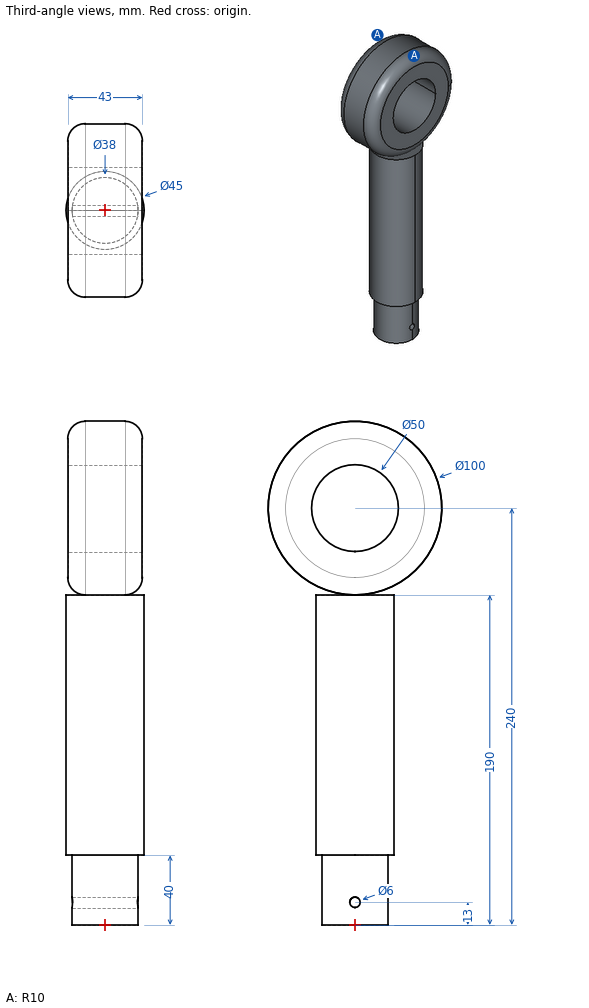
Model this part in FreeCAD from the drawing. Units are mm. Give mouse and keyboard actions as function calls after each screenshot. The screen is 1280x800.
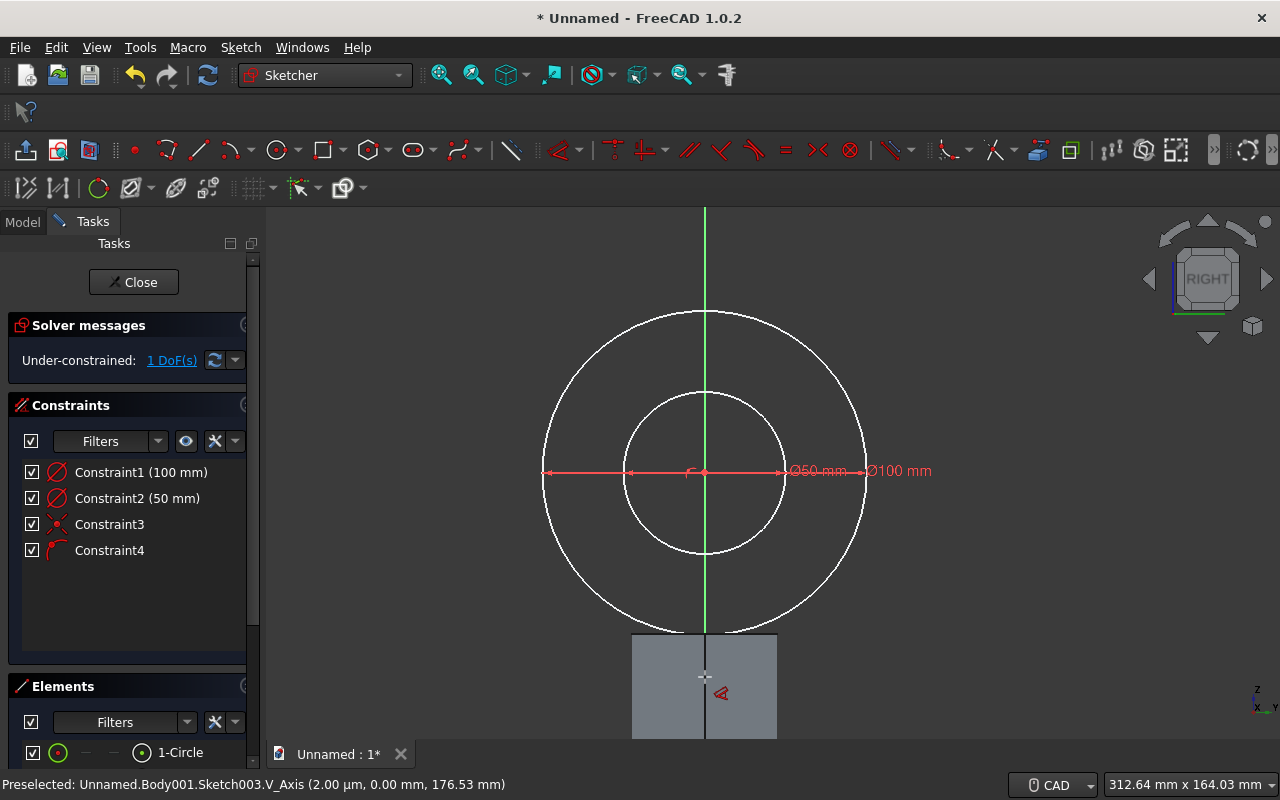
click(705, 473)
click(739, 592)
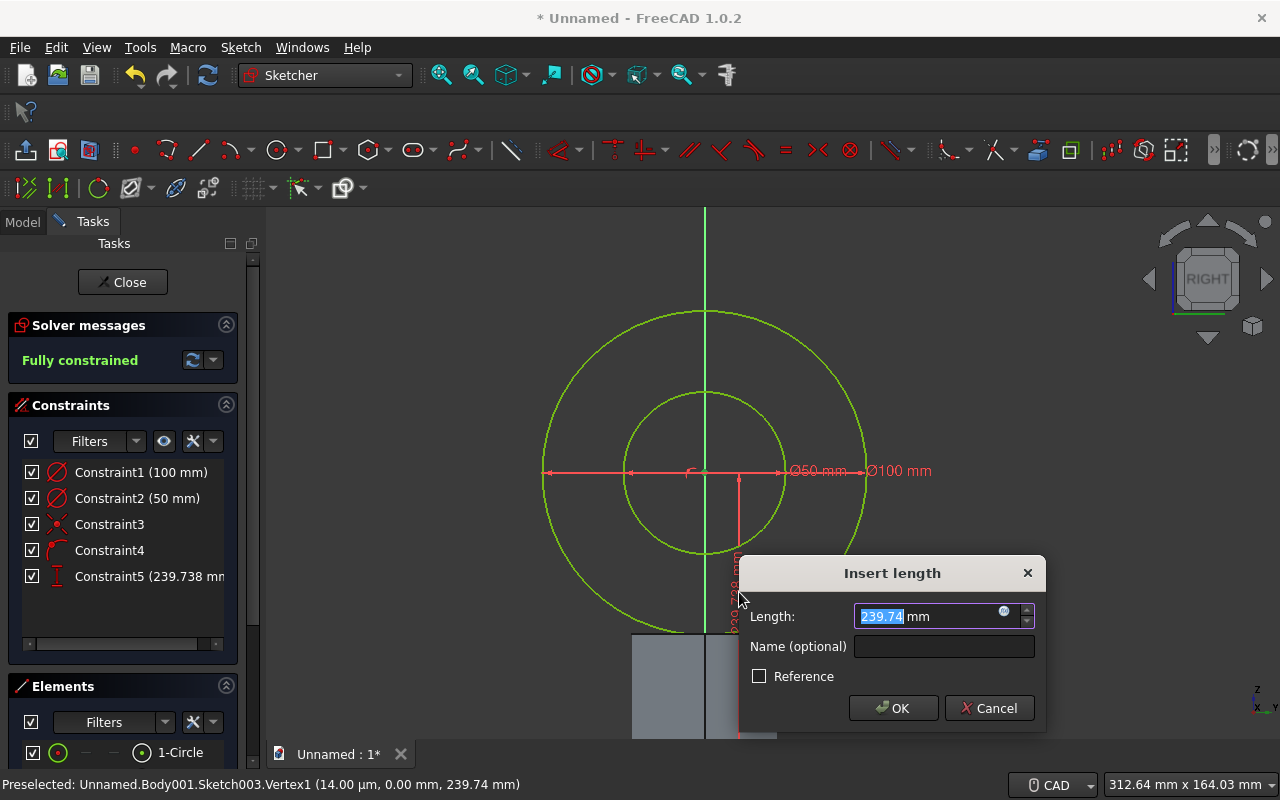
text(240)
key(Return)
key(Escape)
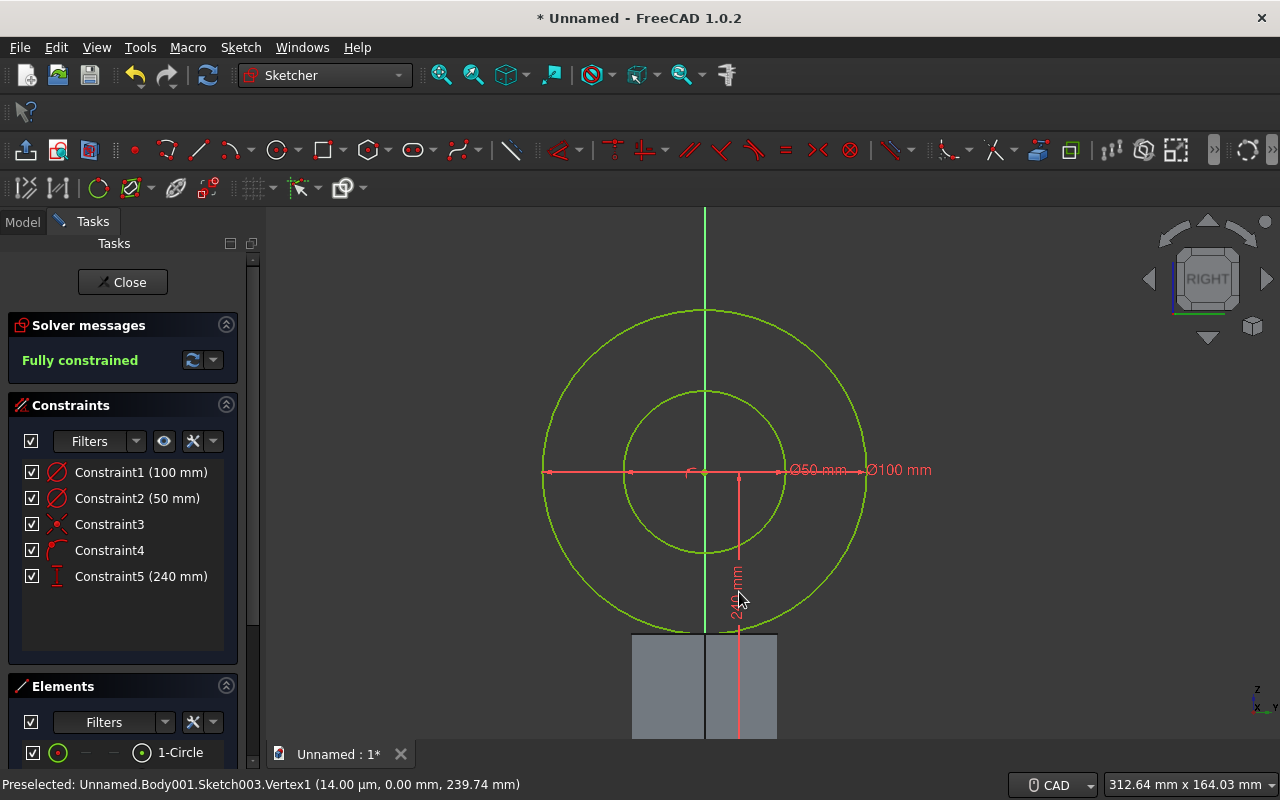
click(123, 282)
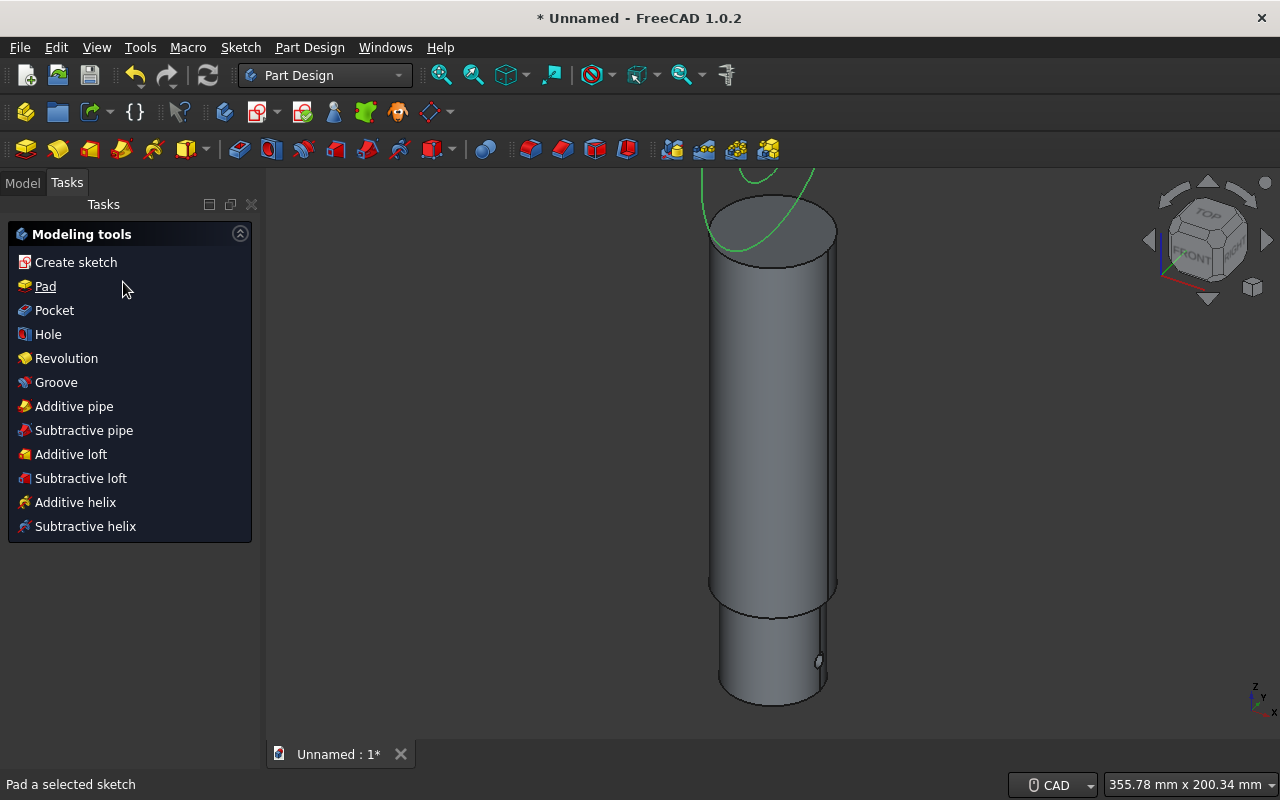
click(26, 150)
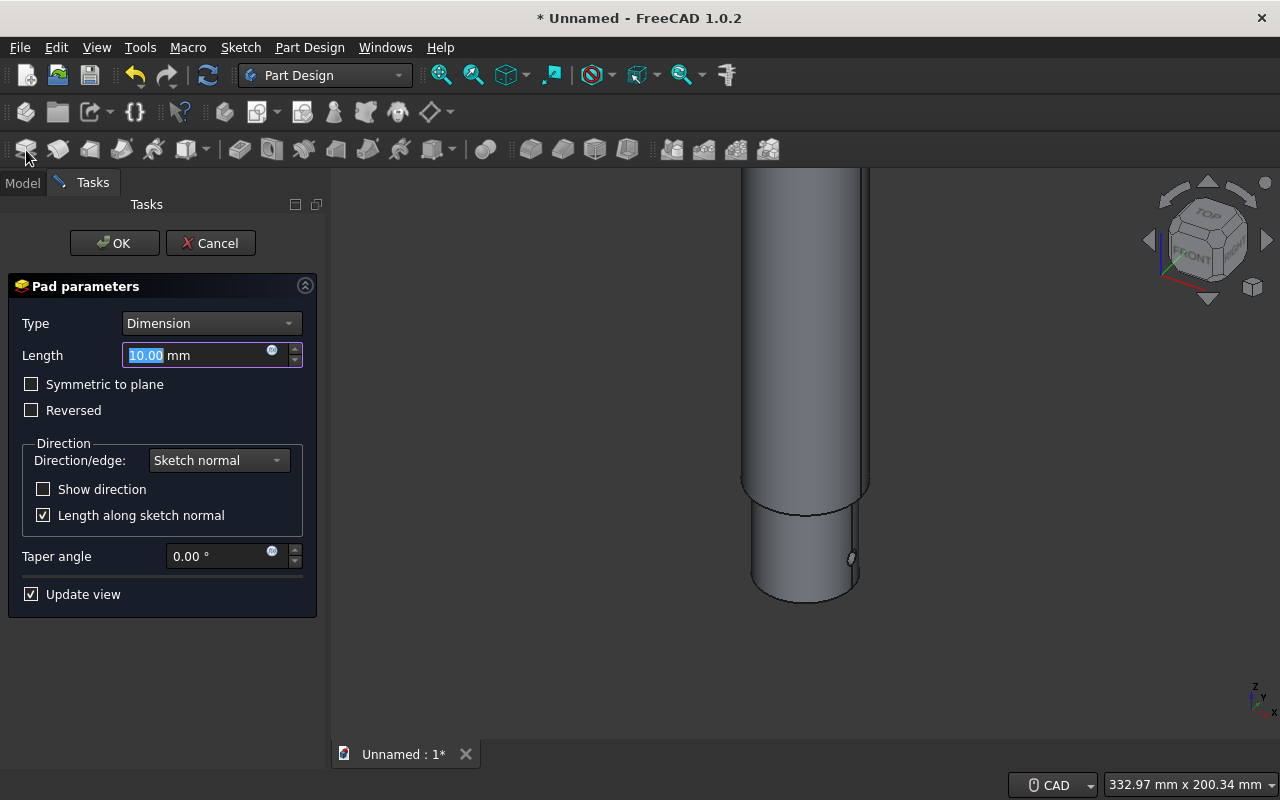
text(43)
key(Tab)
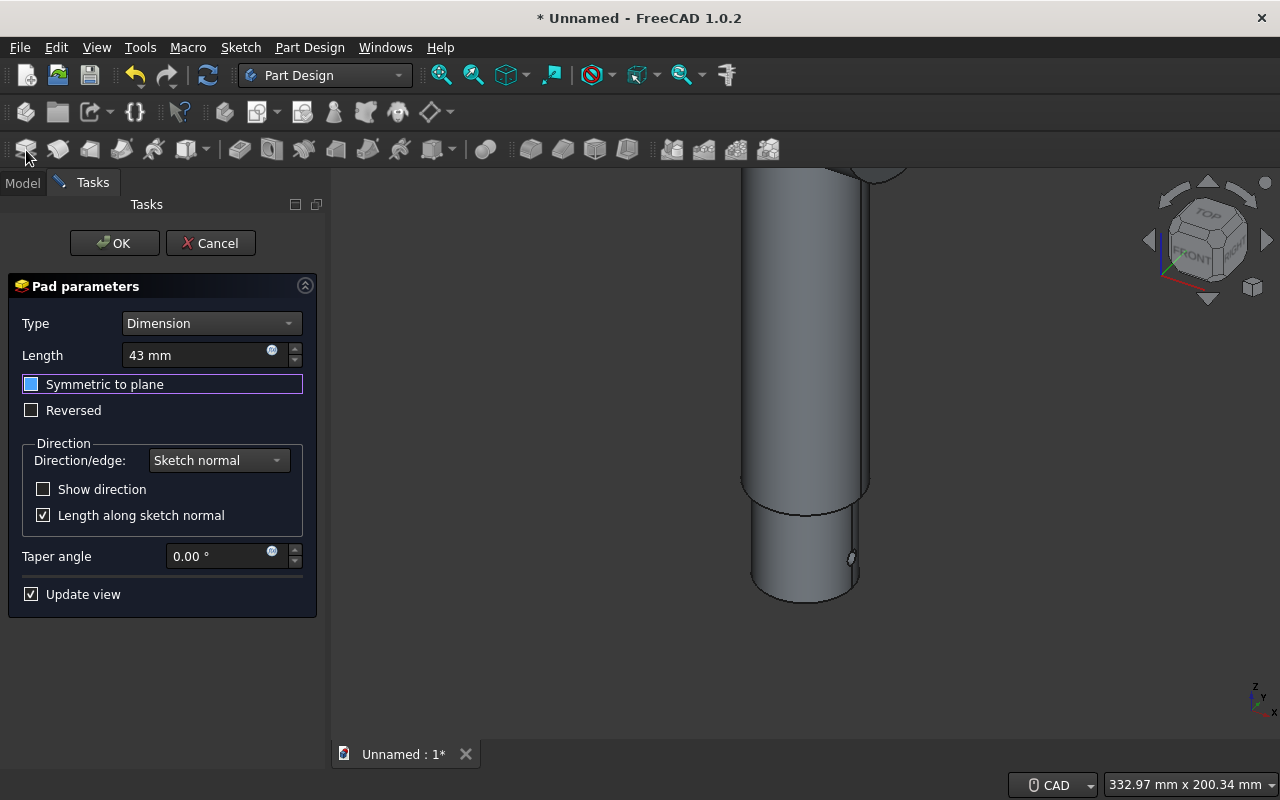
click(30, 384)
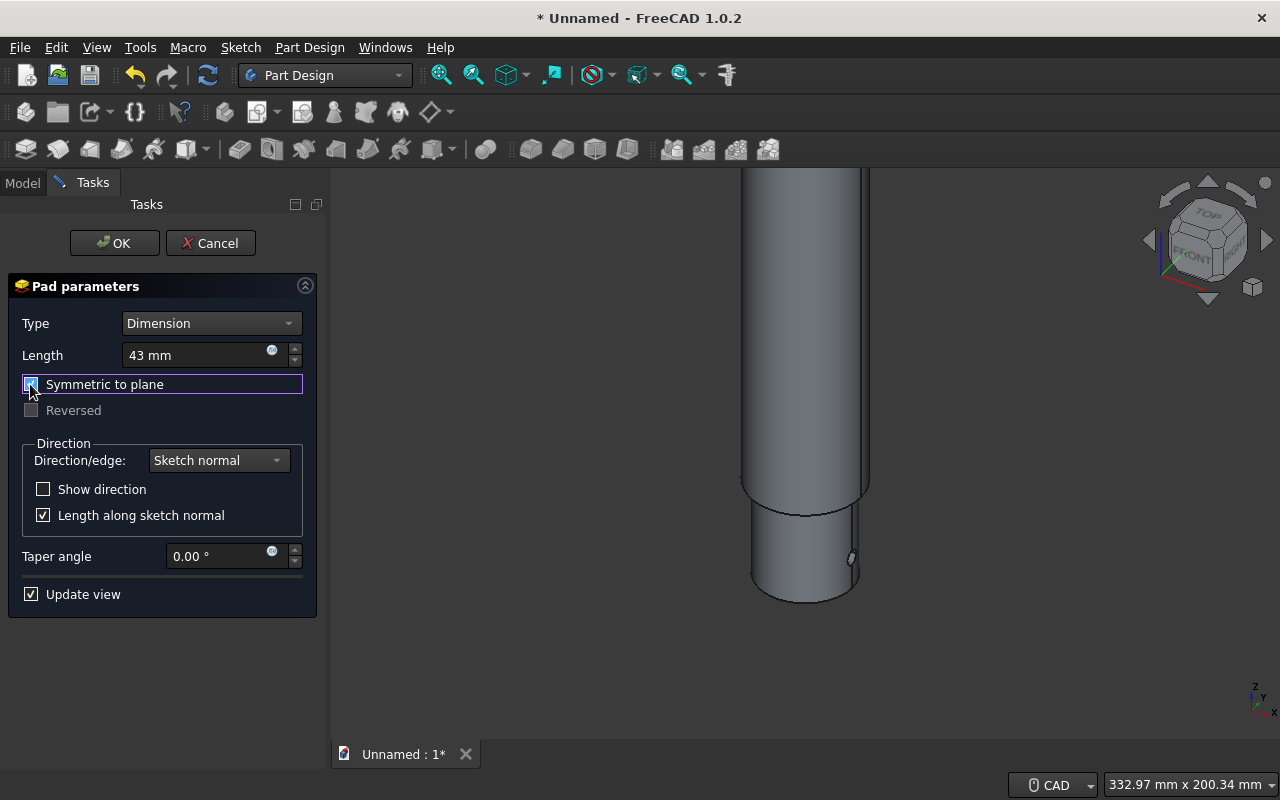
click(115, 243)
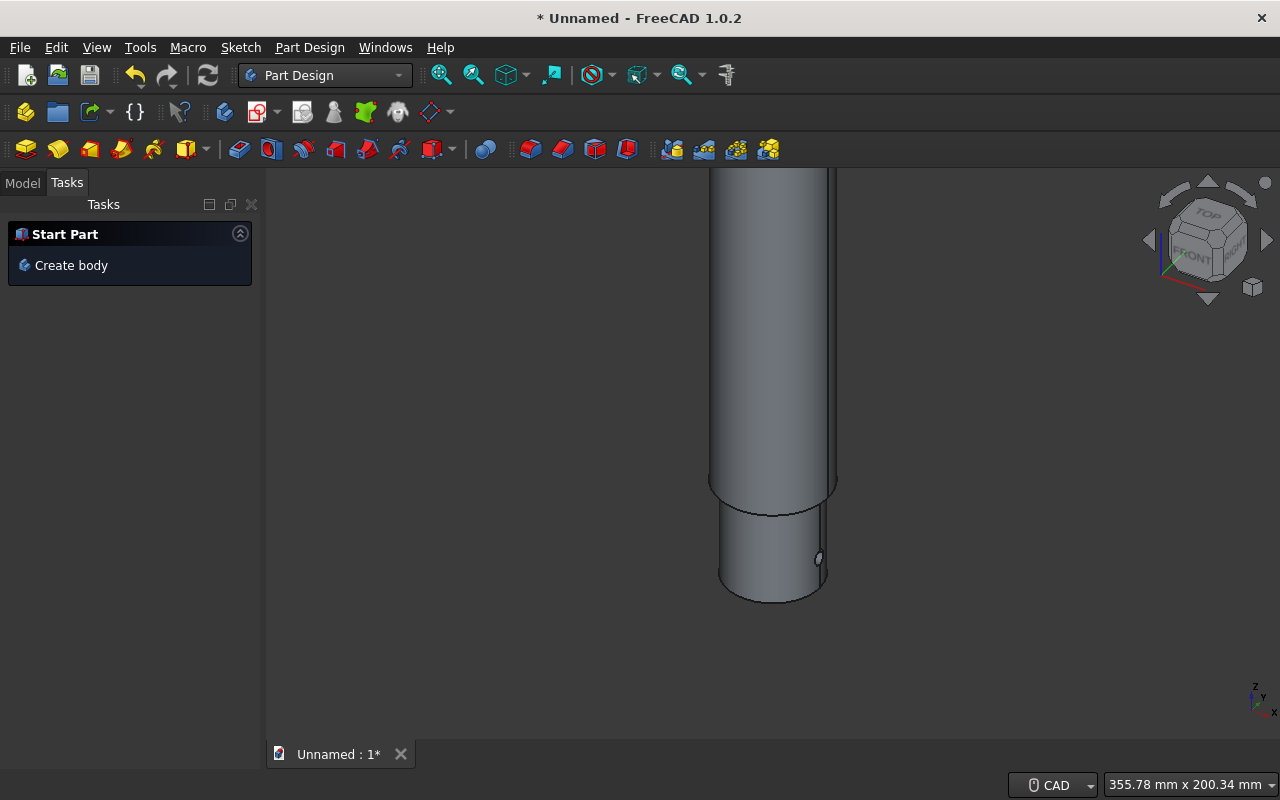
key(v)
key(f)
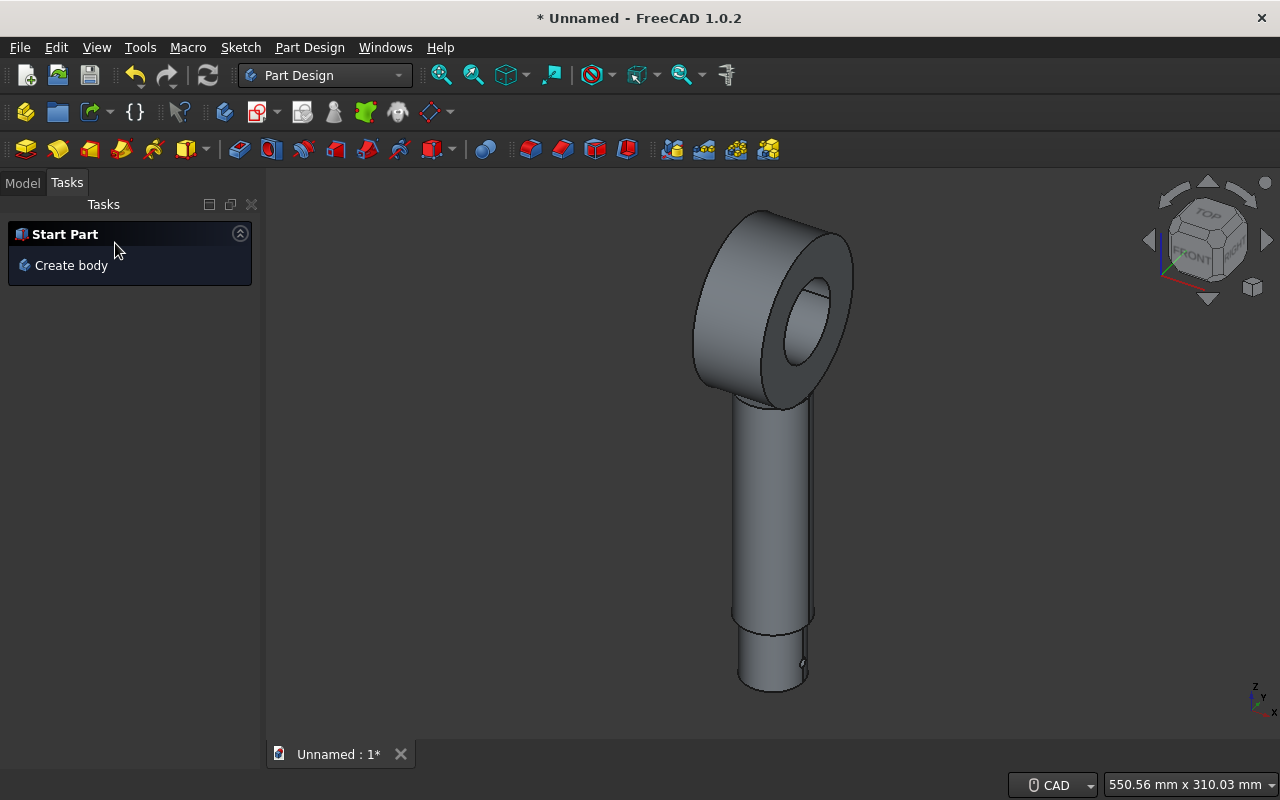
click(701, 379)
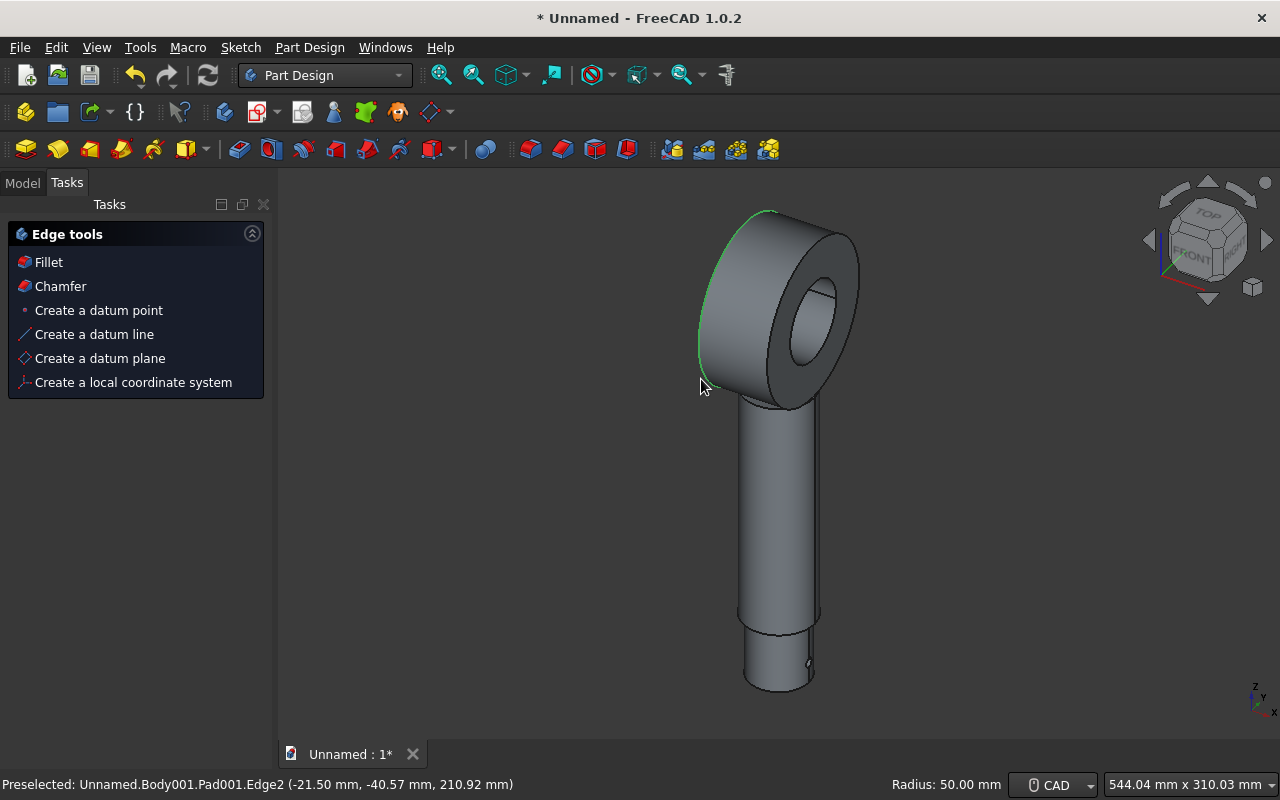
click(767, 366, ctrl)